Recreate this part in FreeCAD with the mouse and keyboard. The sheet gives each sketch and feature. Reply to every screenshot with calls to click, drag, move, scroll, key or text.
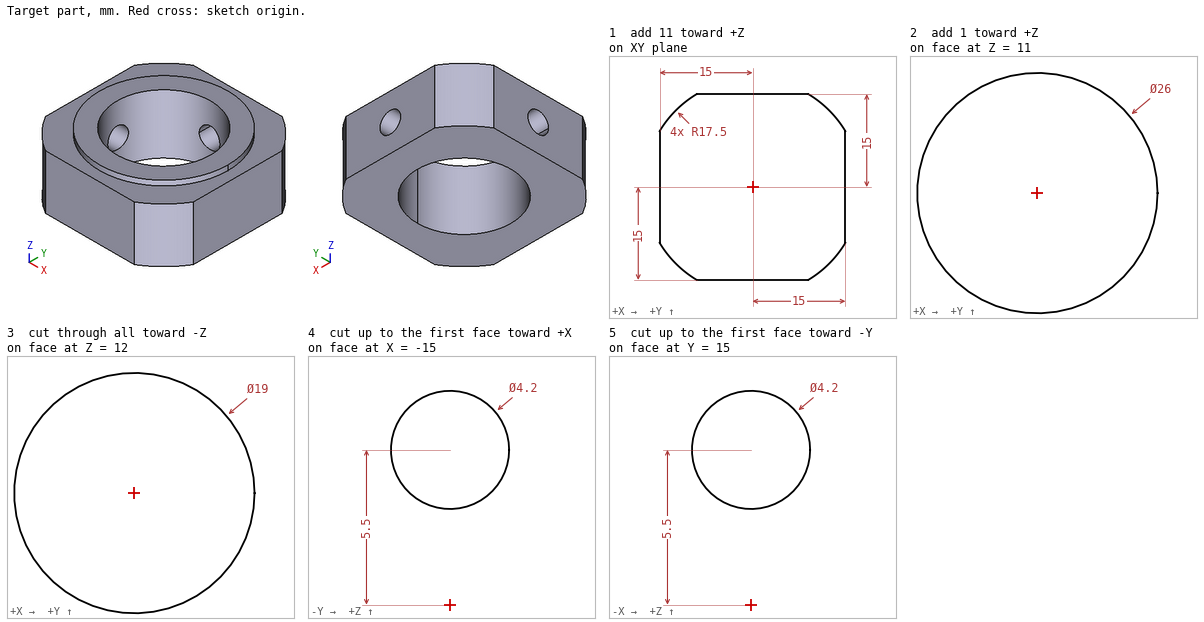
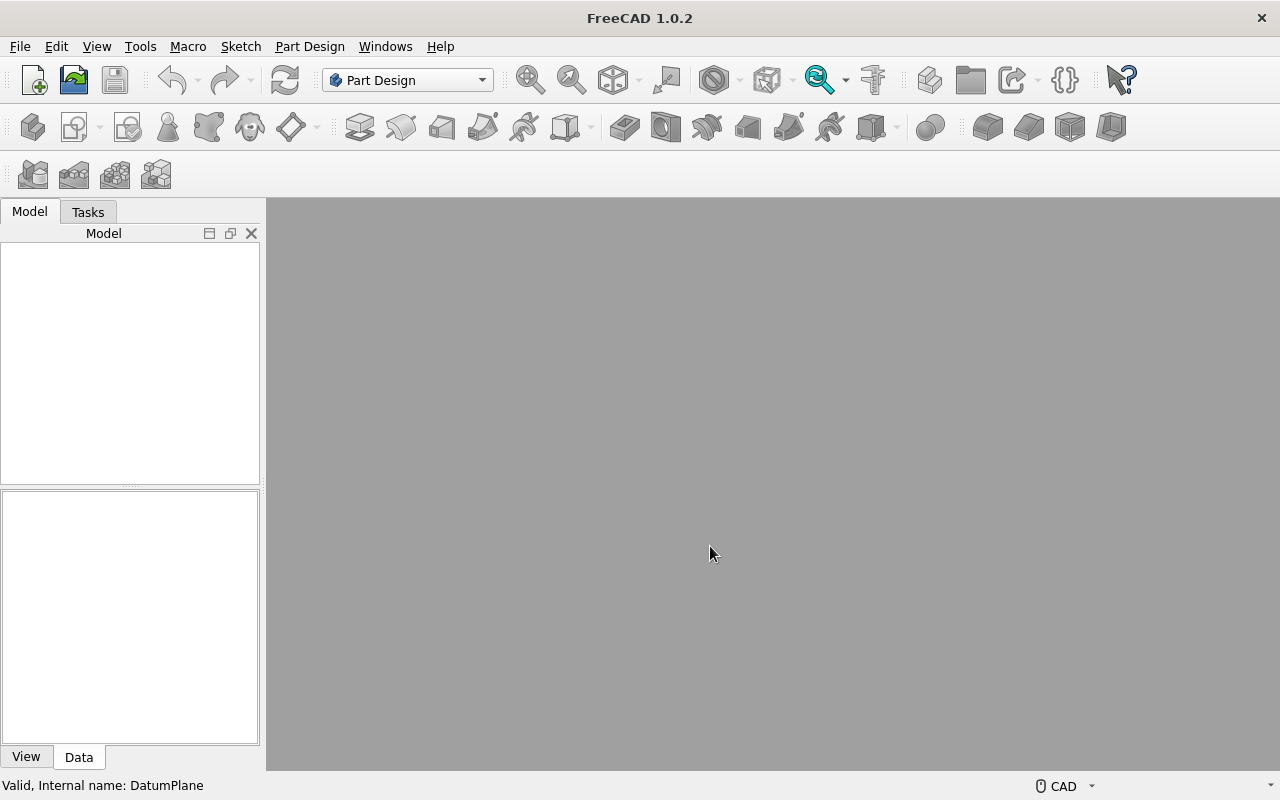
key(ctrl+n)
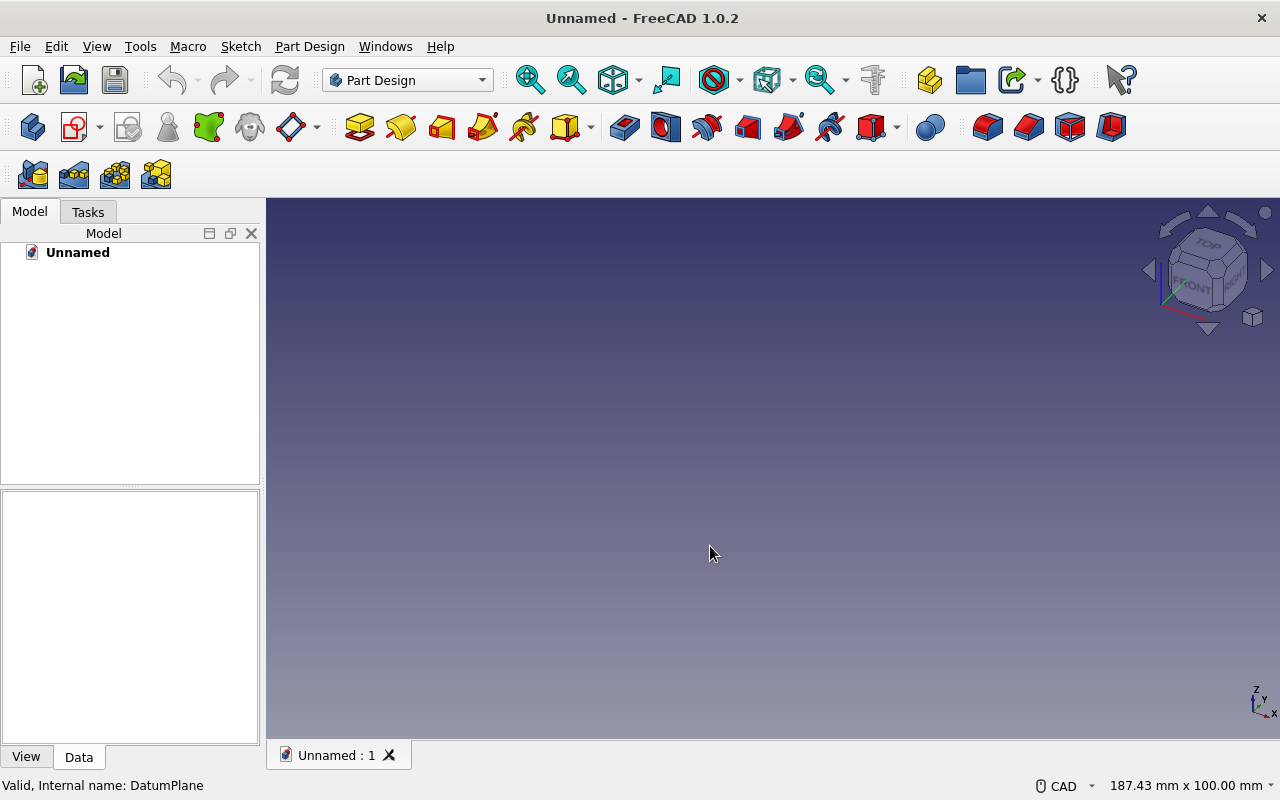
click(74, 128)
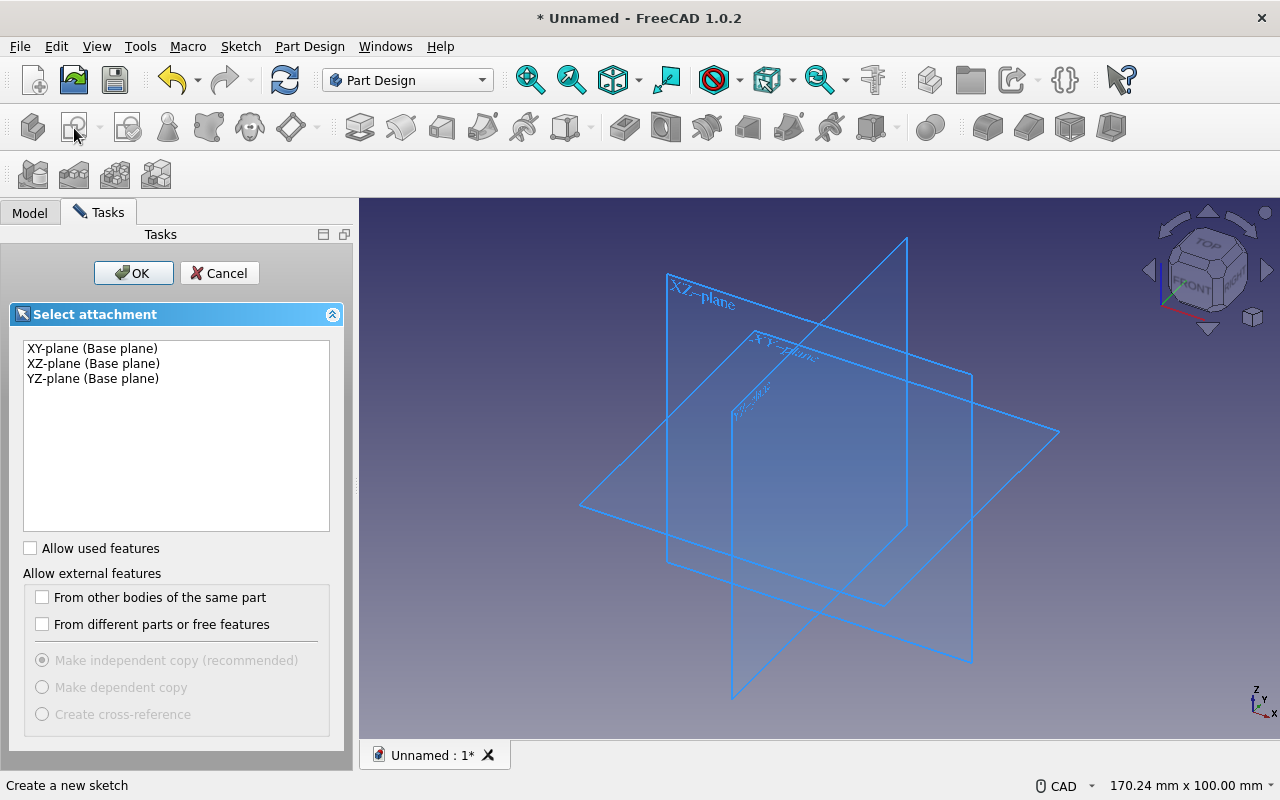
click(84, 348)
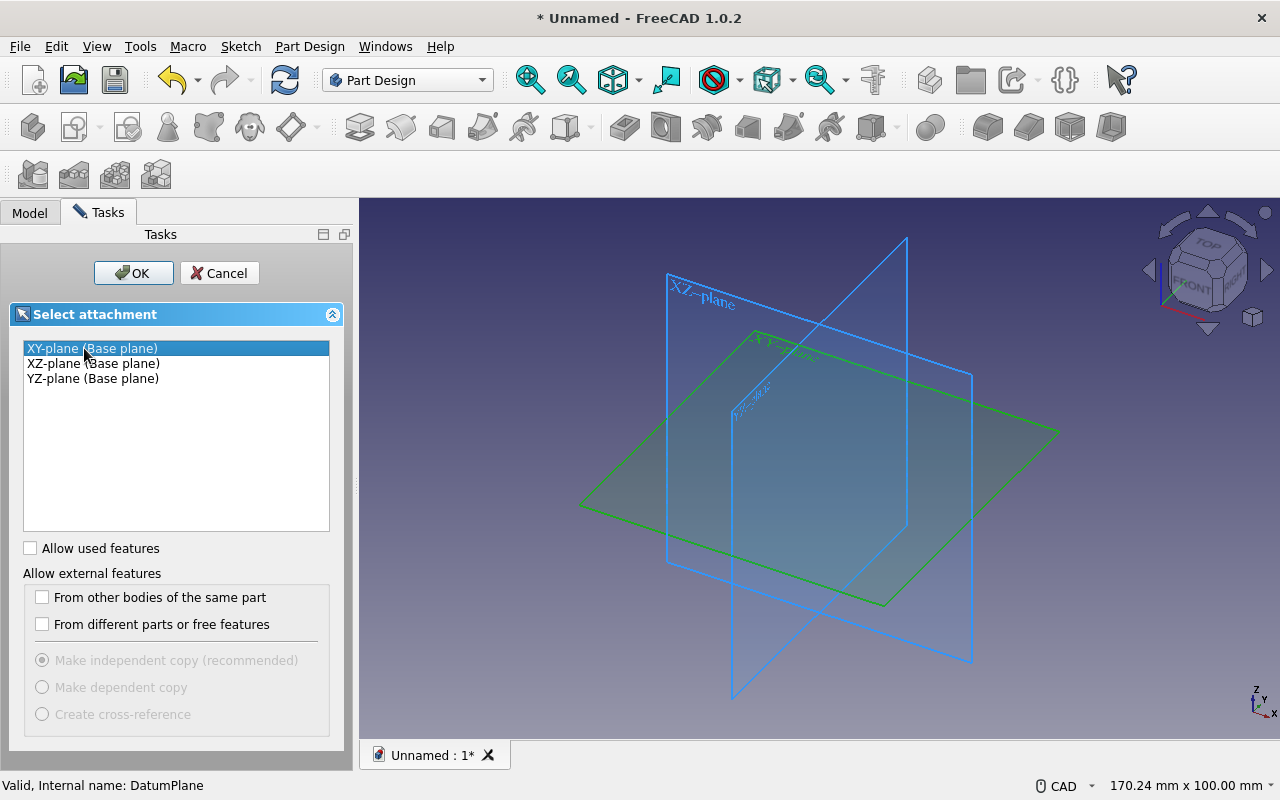
click(134, 273)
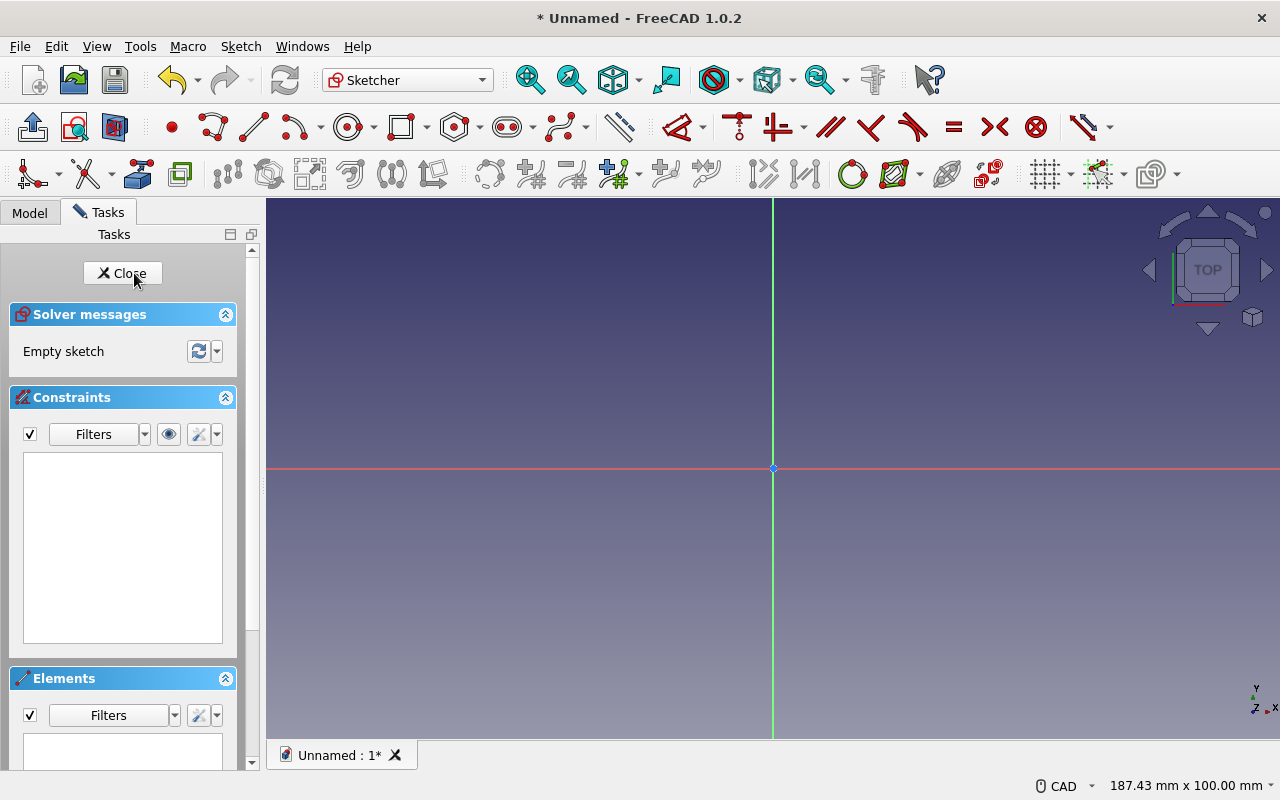
scroll(829, 469, up, 4)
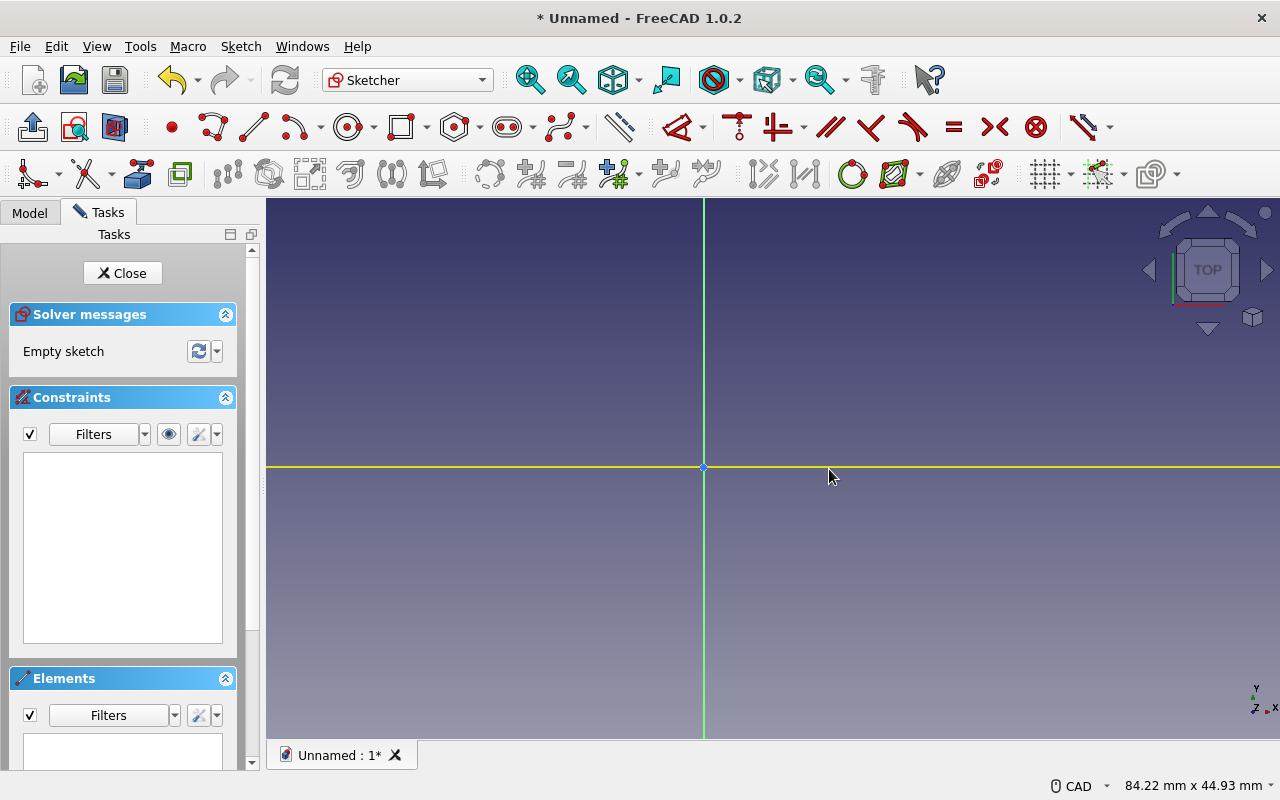
click(254, 128)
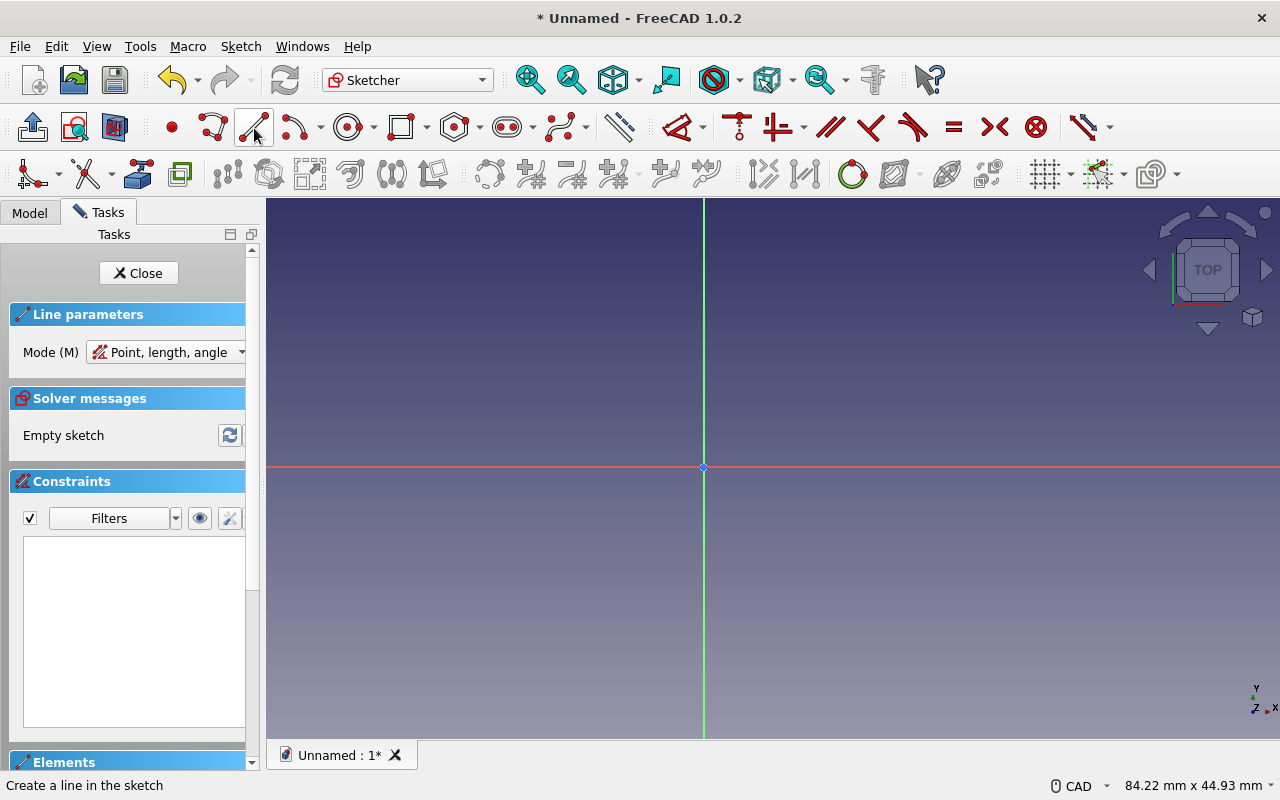
click(812, 287)
click(595, 287)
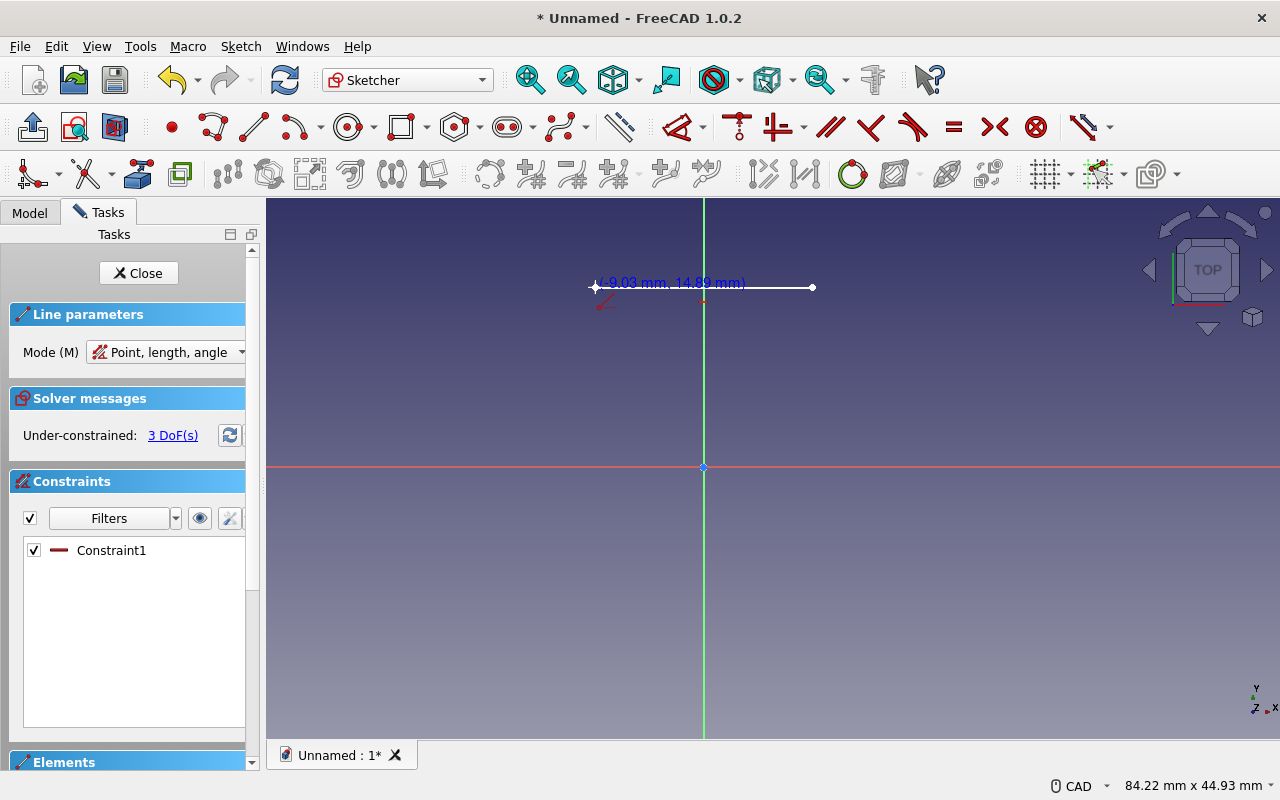
click(523, 359)
click(523, 576)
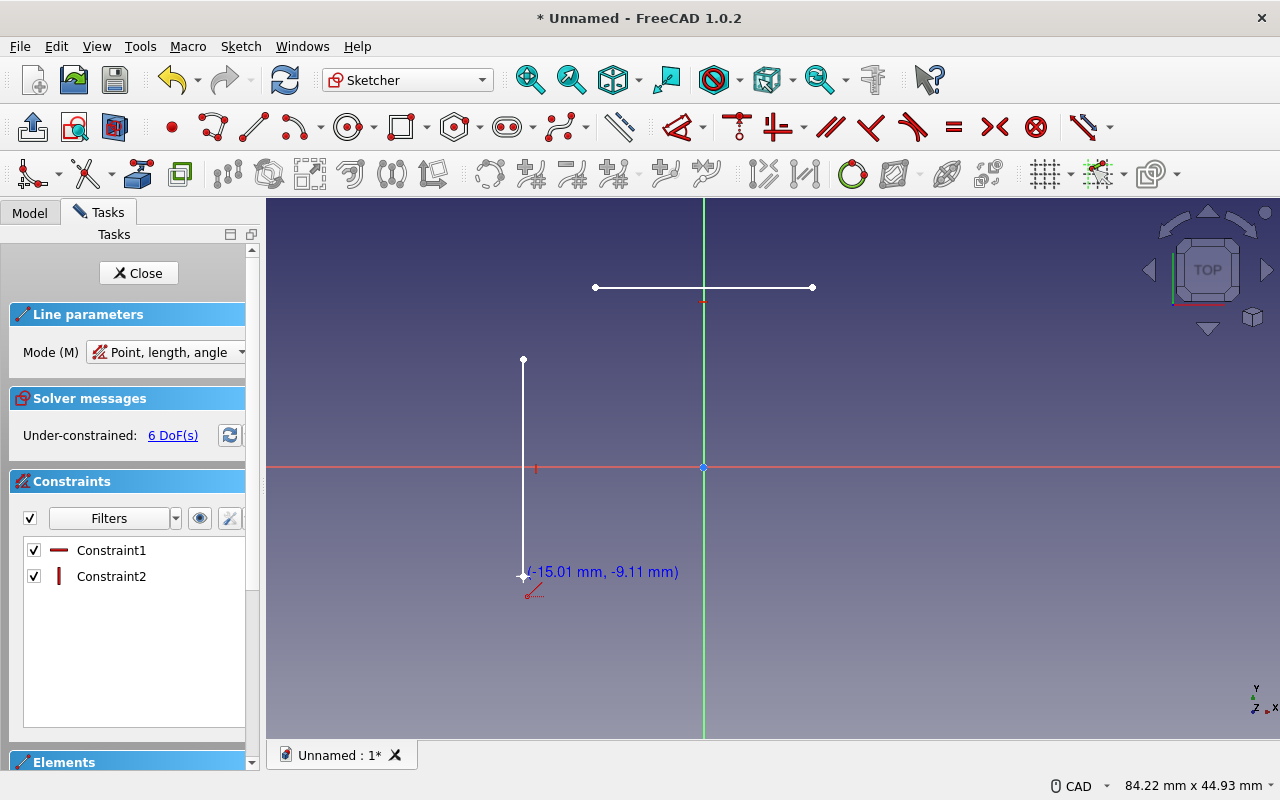
click(595, 648)
click(812, 648)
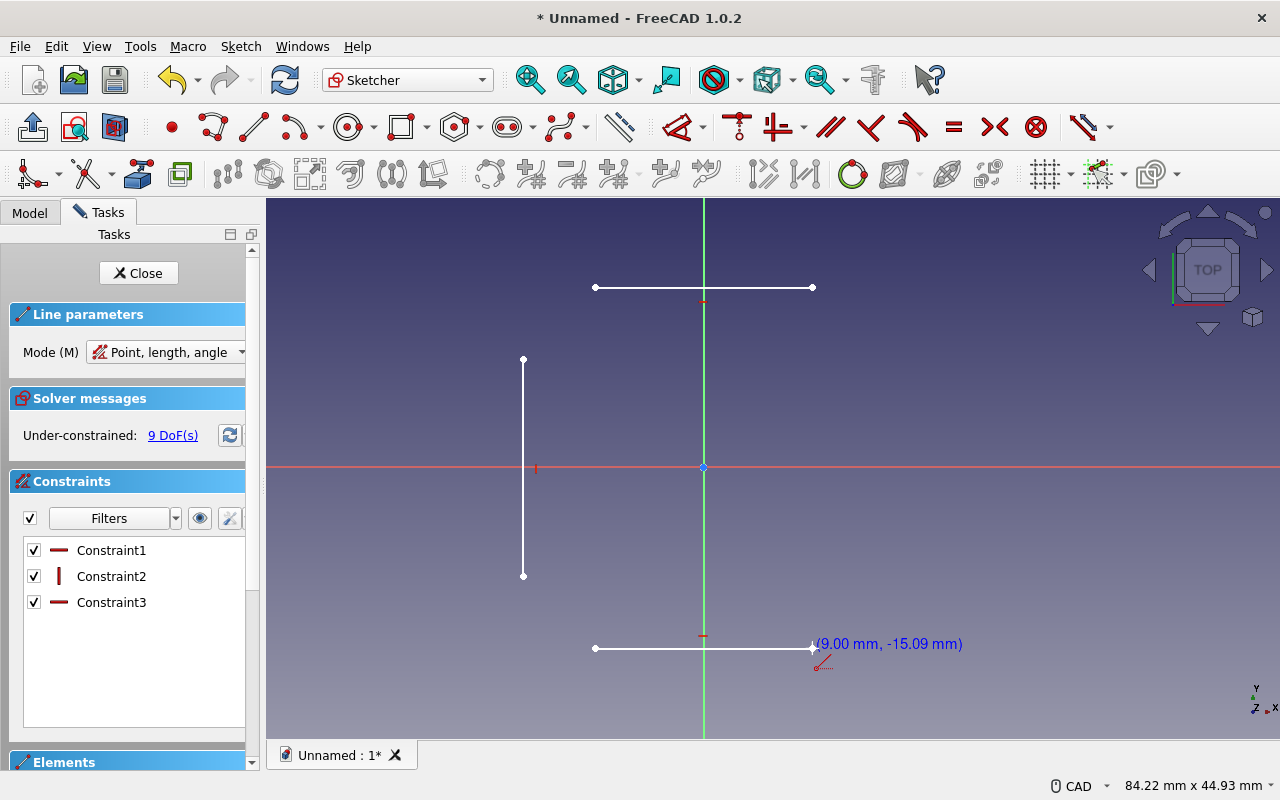
click(884, 576)
click(884, 359)